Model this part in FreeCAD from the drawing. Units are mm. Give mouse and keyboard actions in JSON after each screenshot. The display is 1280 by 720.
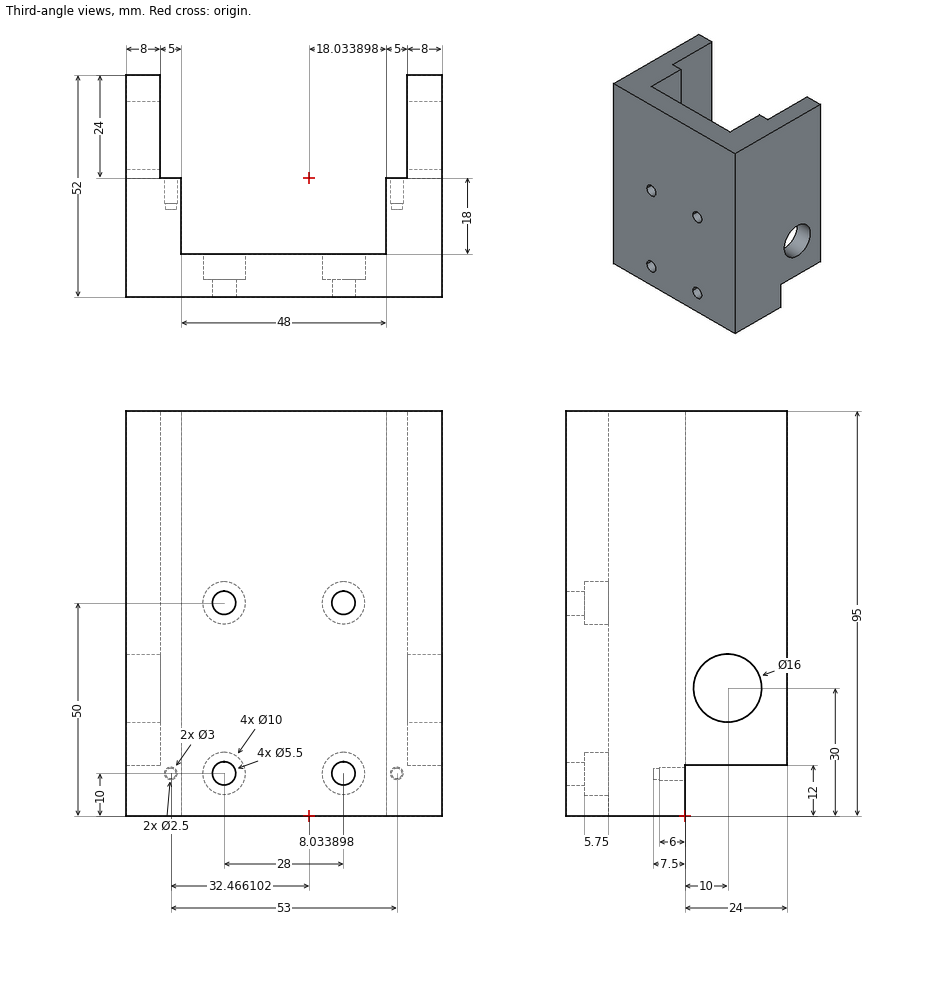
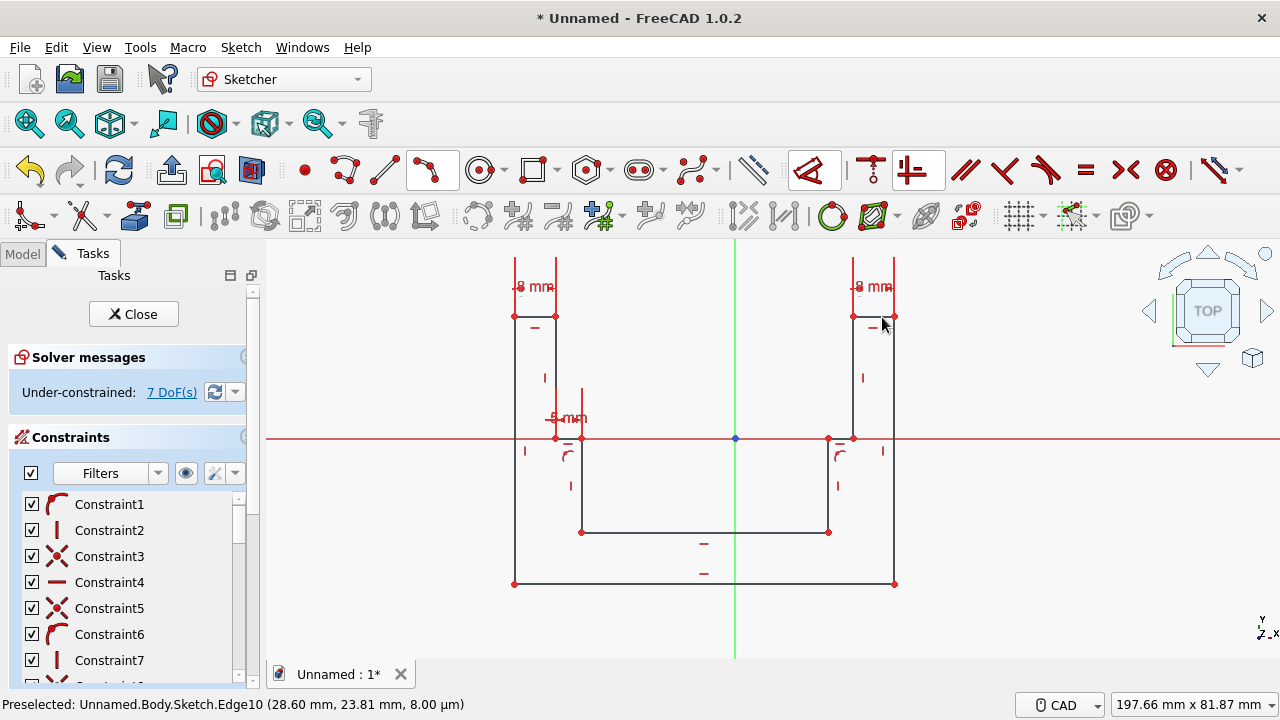
{"action": "scroll", "coordinate": [843, 439], "scroll_direction": "up", "scroll_amount": 3}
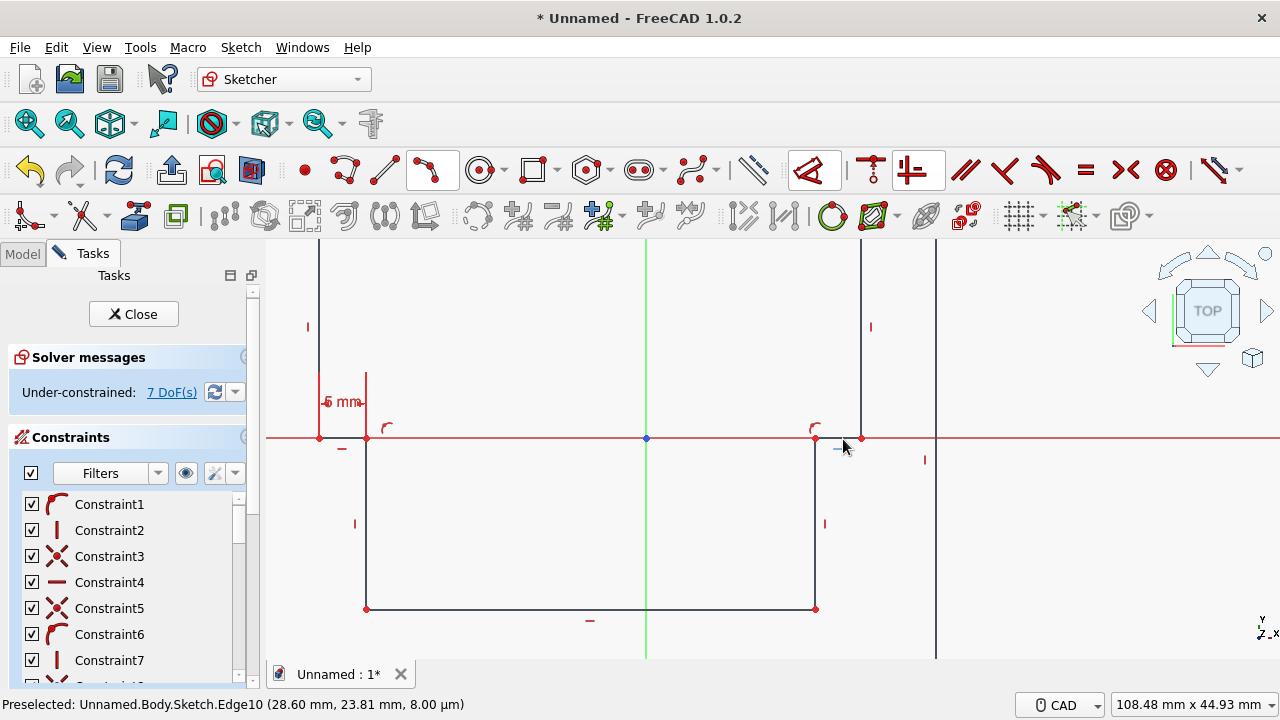
{"action": "left_click", "coordinate": [843, 438]}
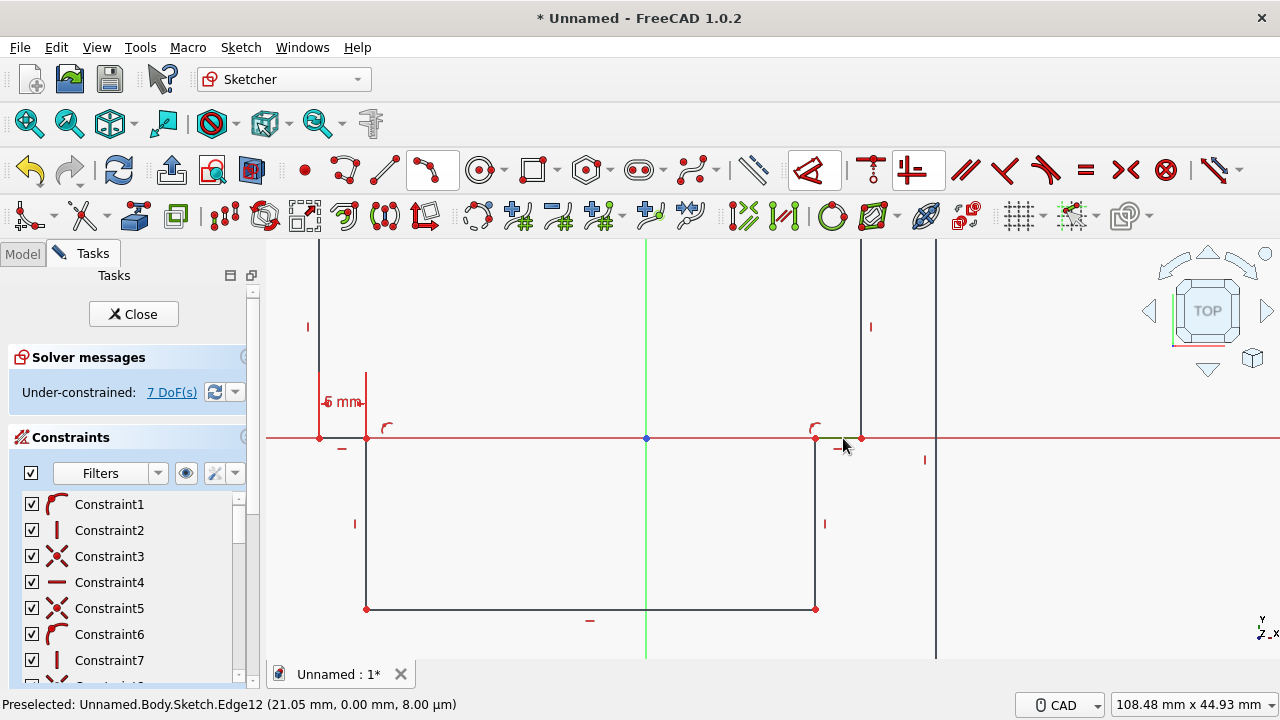
{"action": "key", "text": "l"}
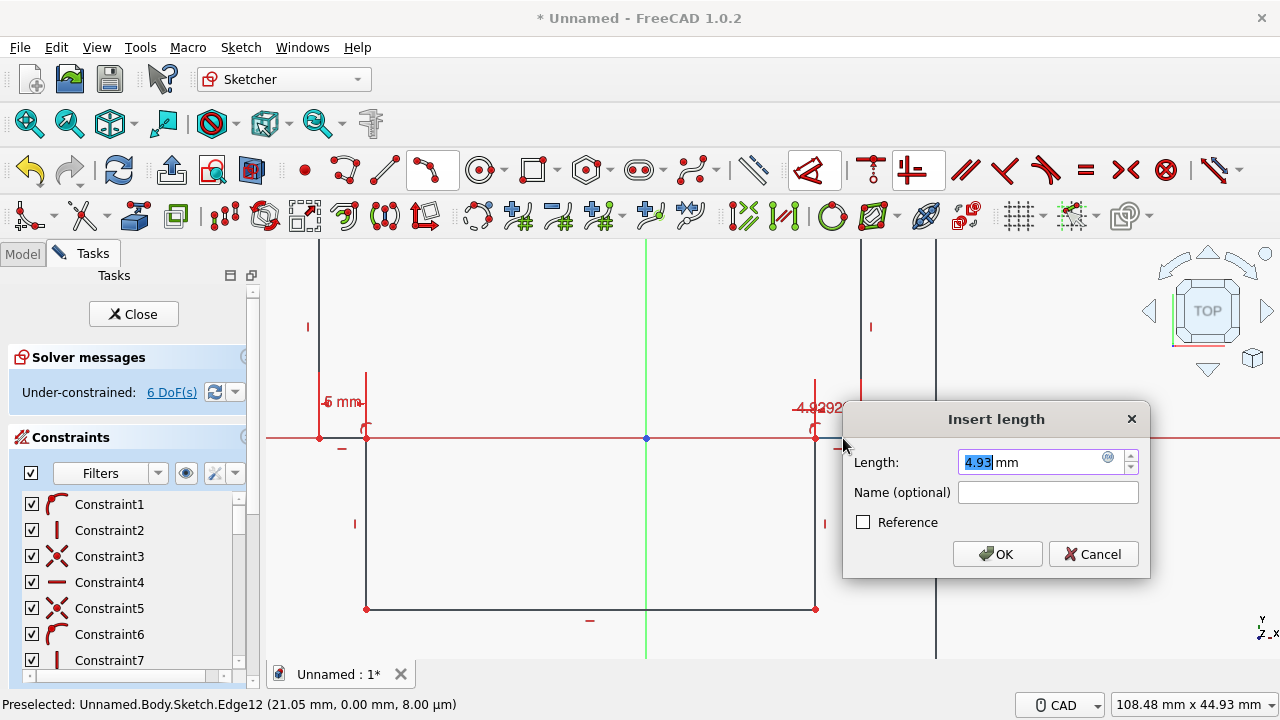
{"action": "type", "text": "5"}
{"action": "key", "text": "Return"}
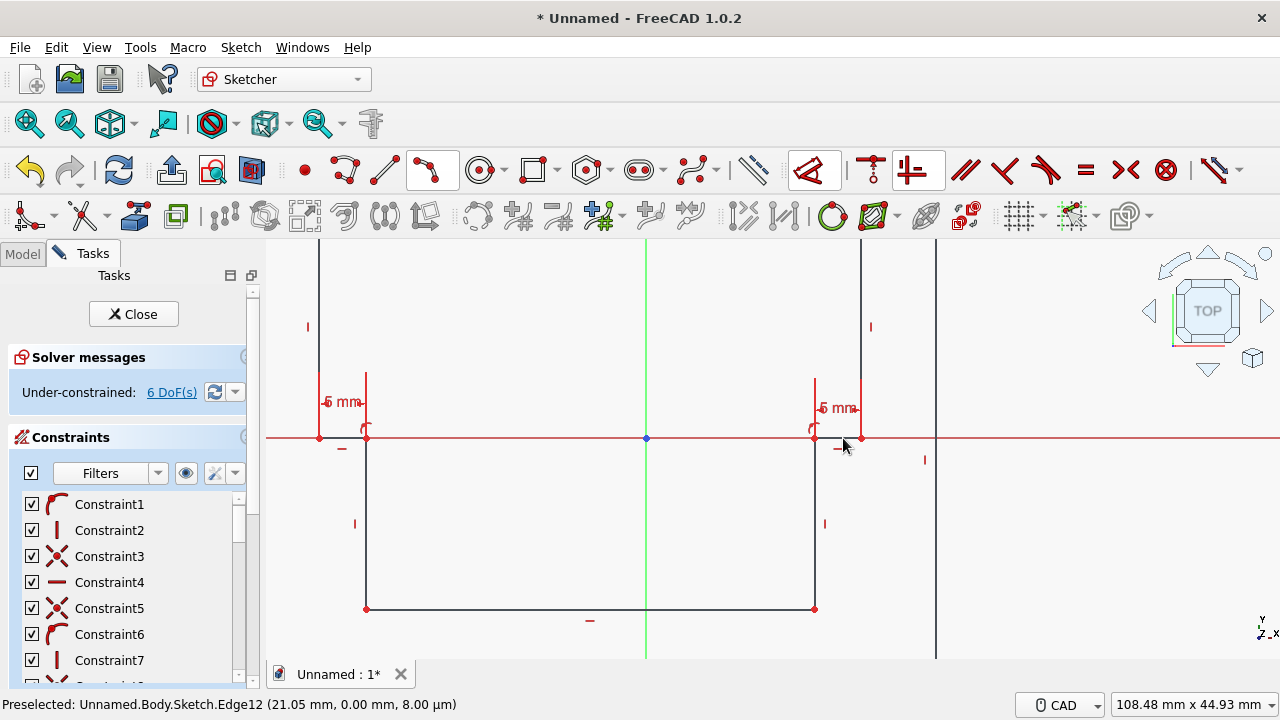
{"action": "left_click", "coordinate": [815, 490]}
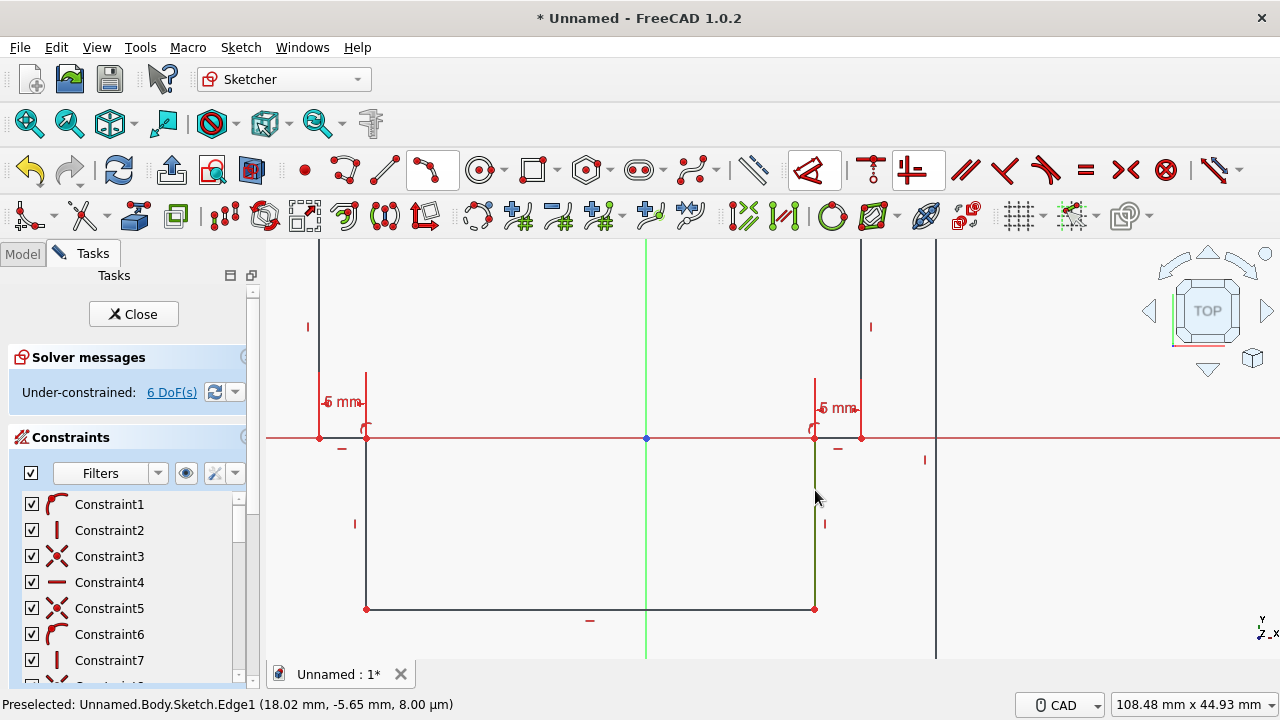
{"action": "left_click", "coordinate": [836, 170]}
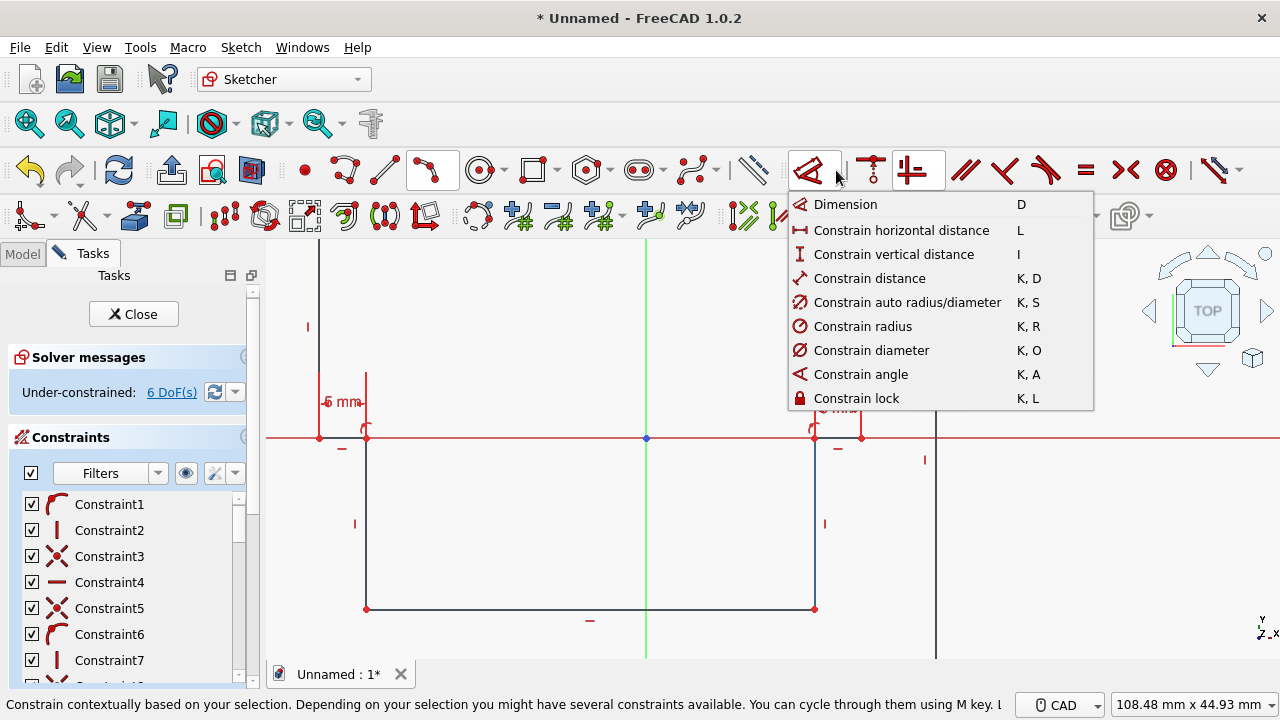
{"action": "left_click", "coordinate": [941, 254]}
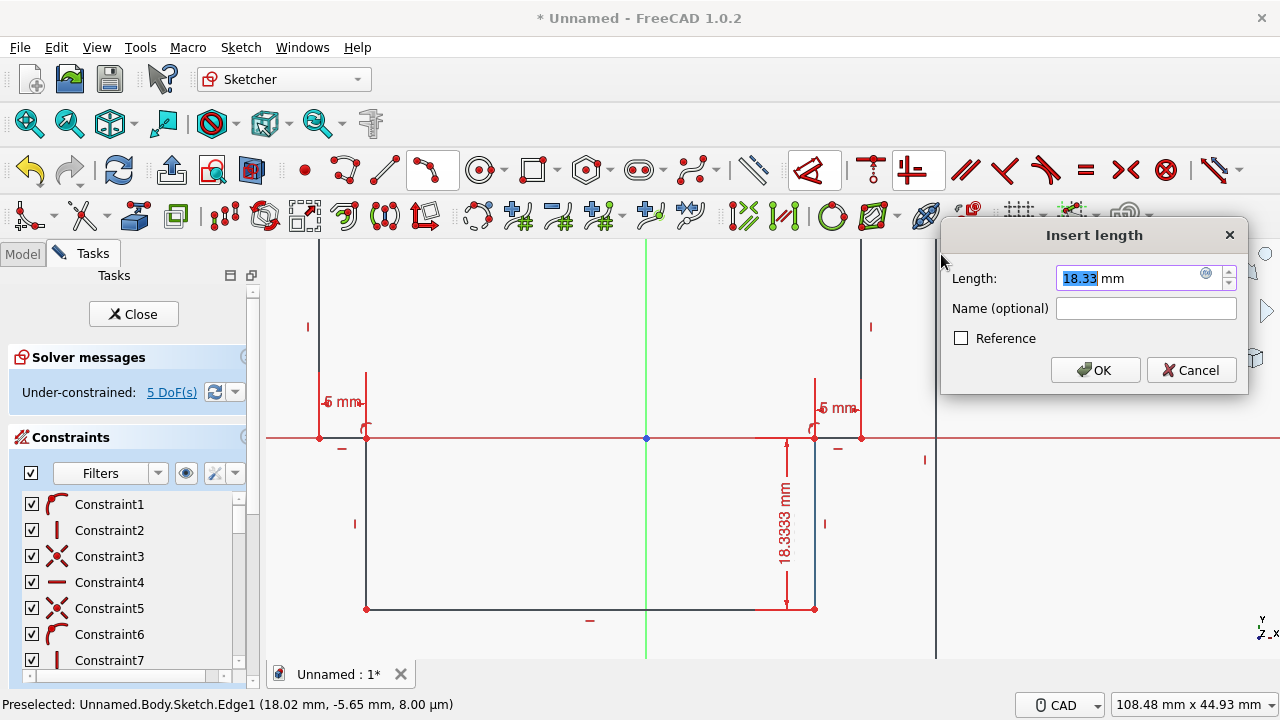
{"action": "type", "text": "18"}
{"action": "key", "text": "Return"}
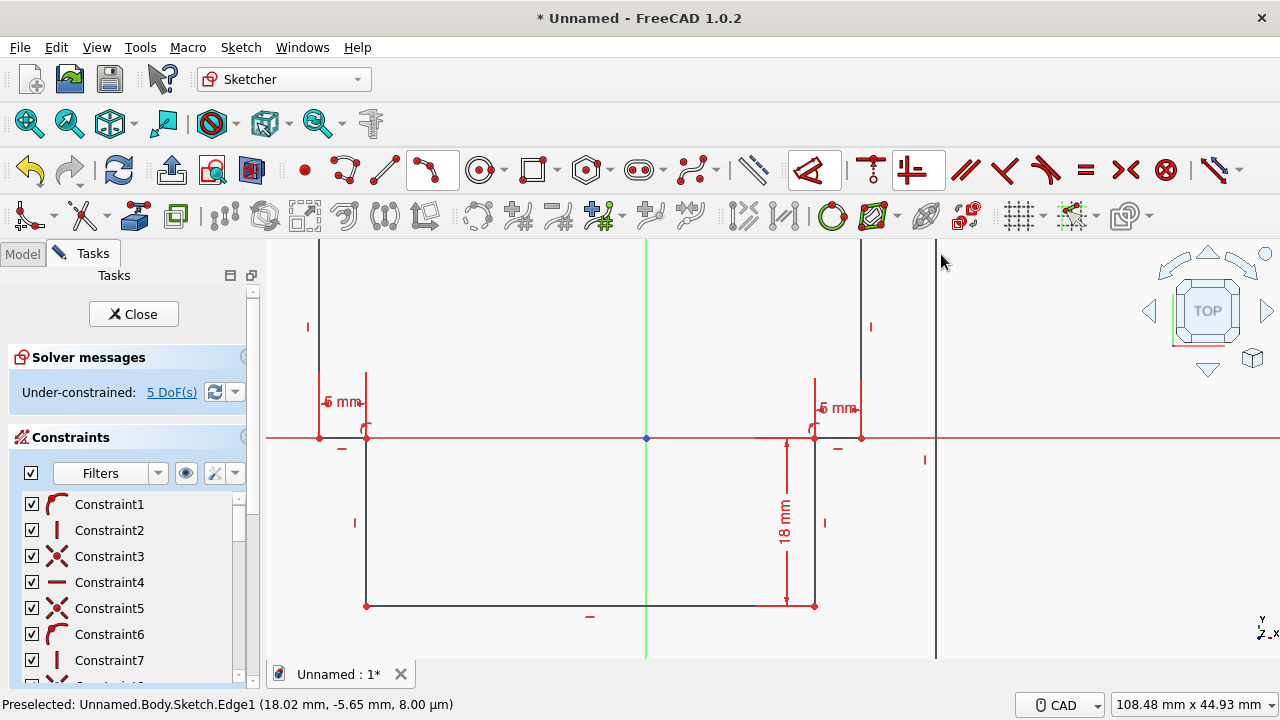
{"action": "left_click", "coordinate": [680, 606]}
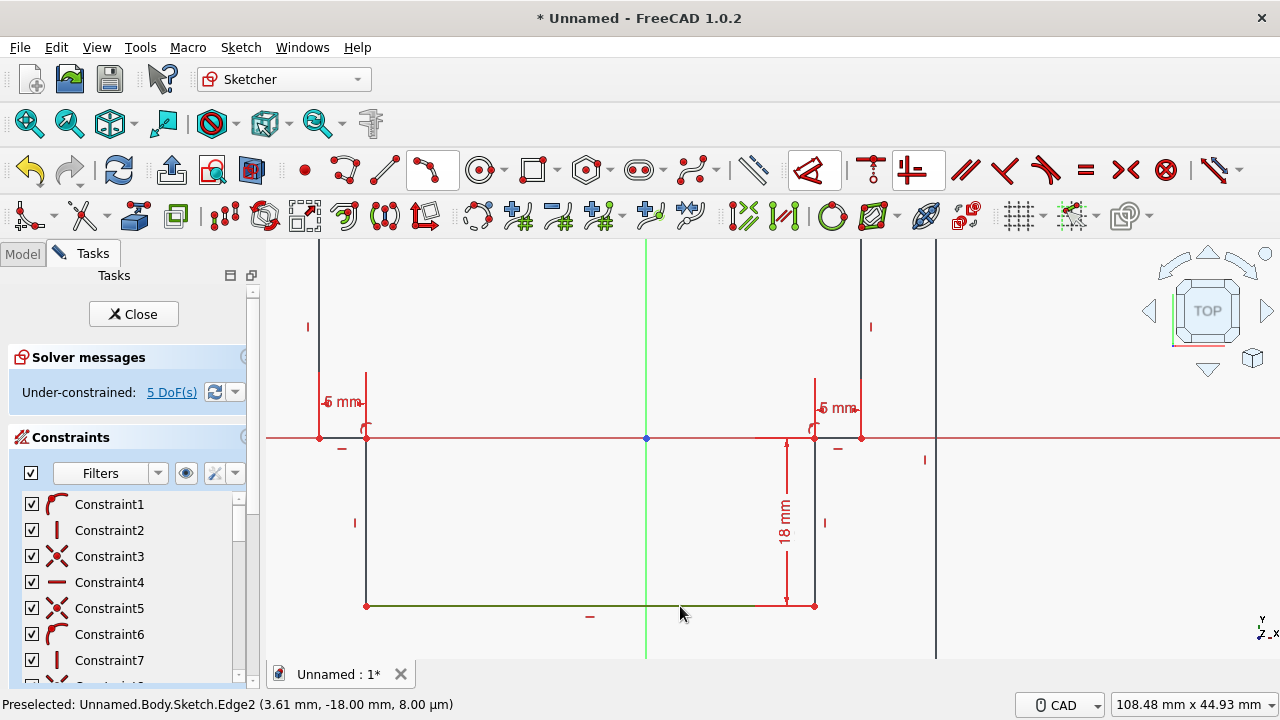
{"action": "key", "text": "l"}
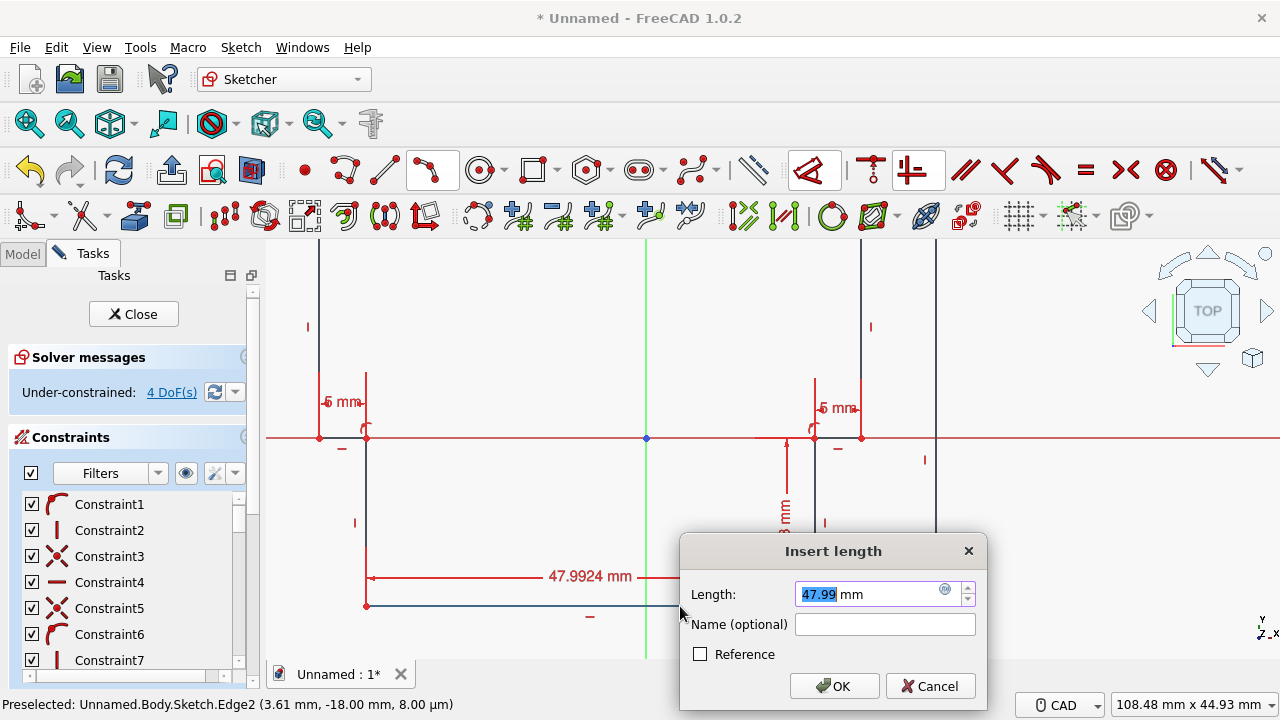
{"action": "type", "text": "48"}
{"action": "key", "text": "Return"}